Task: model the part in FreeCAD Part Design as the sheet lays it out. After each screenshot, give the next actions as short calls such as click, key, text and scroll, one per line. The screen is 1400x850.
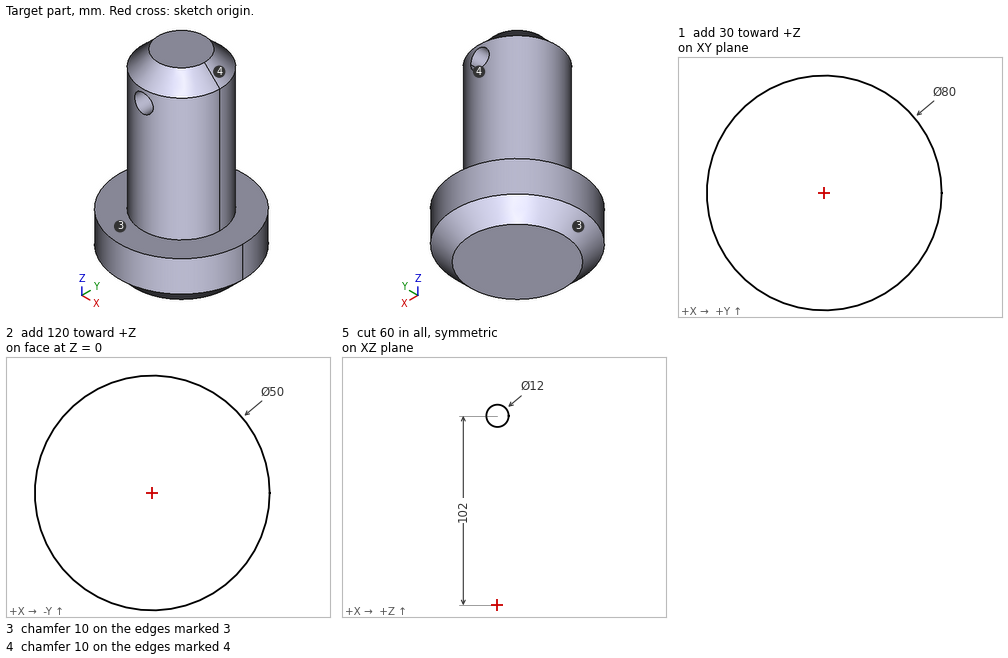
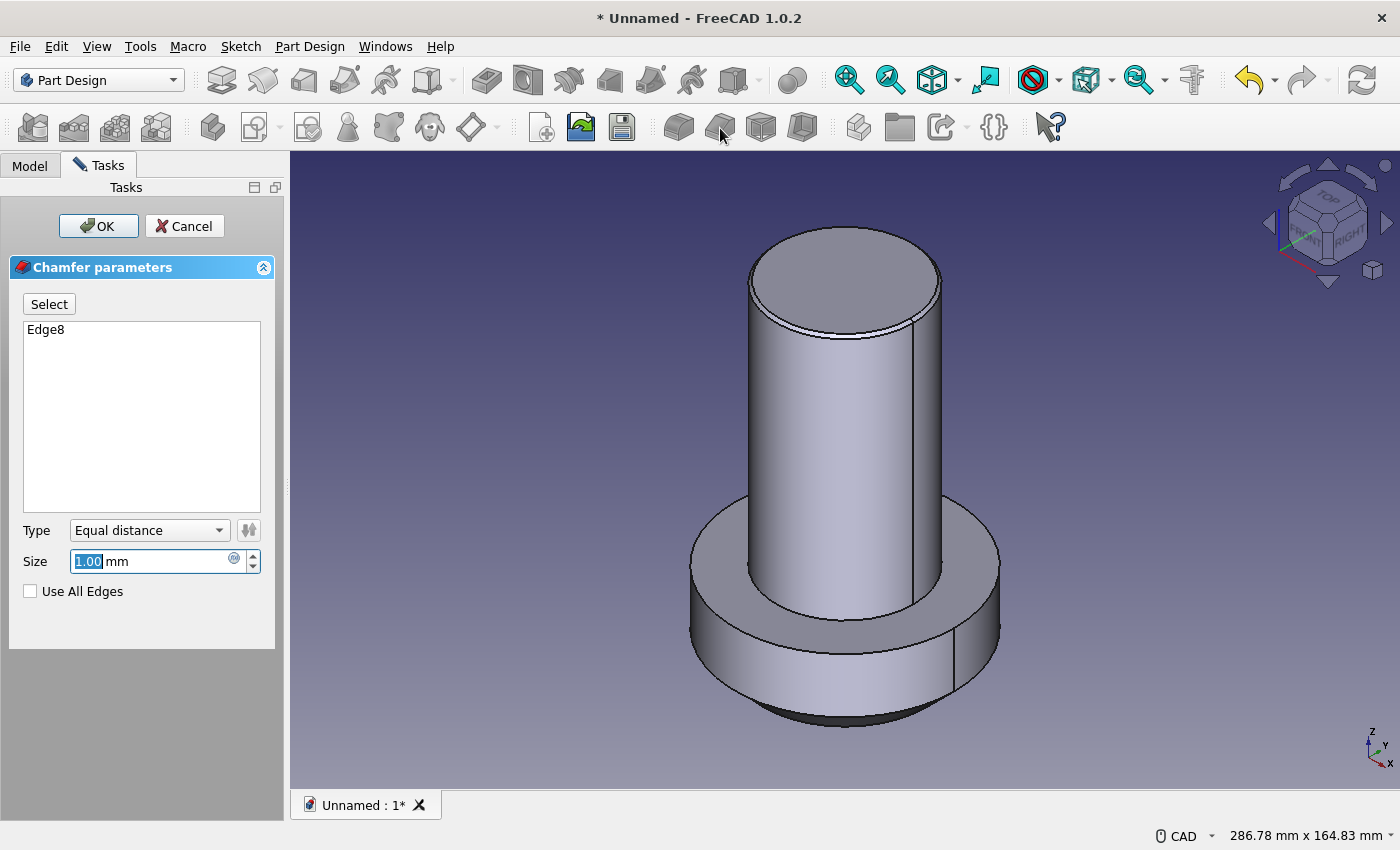
text(10)
key(Tab)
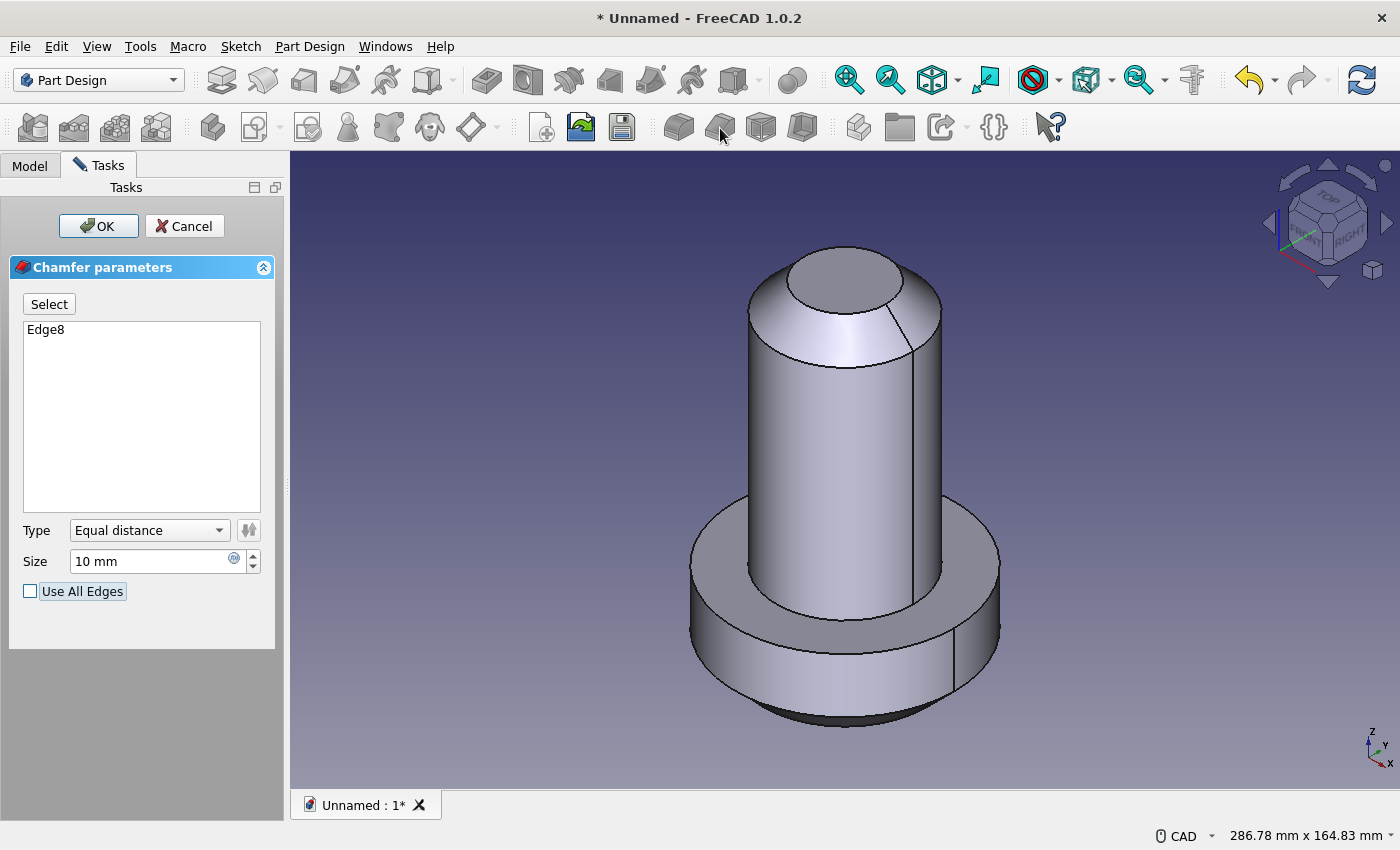
click(99, 226)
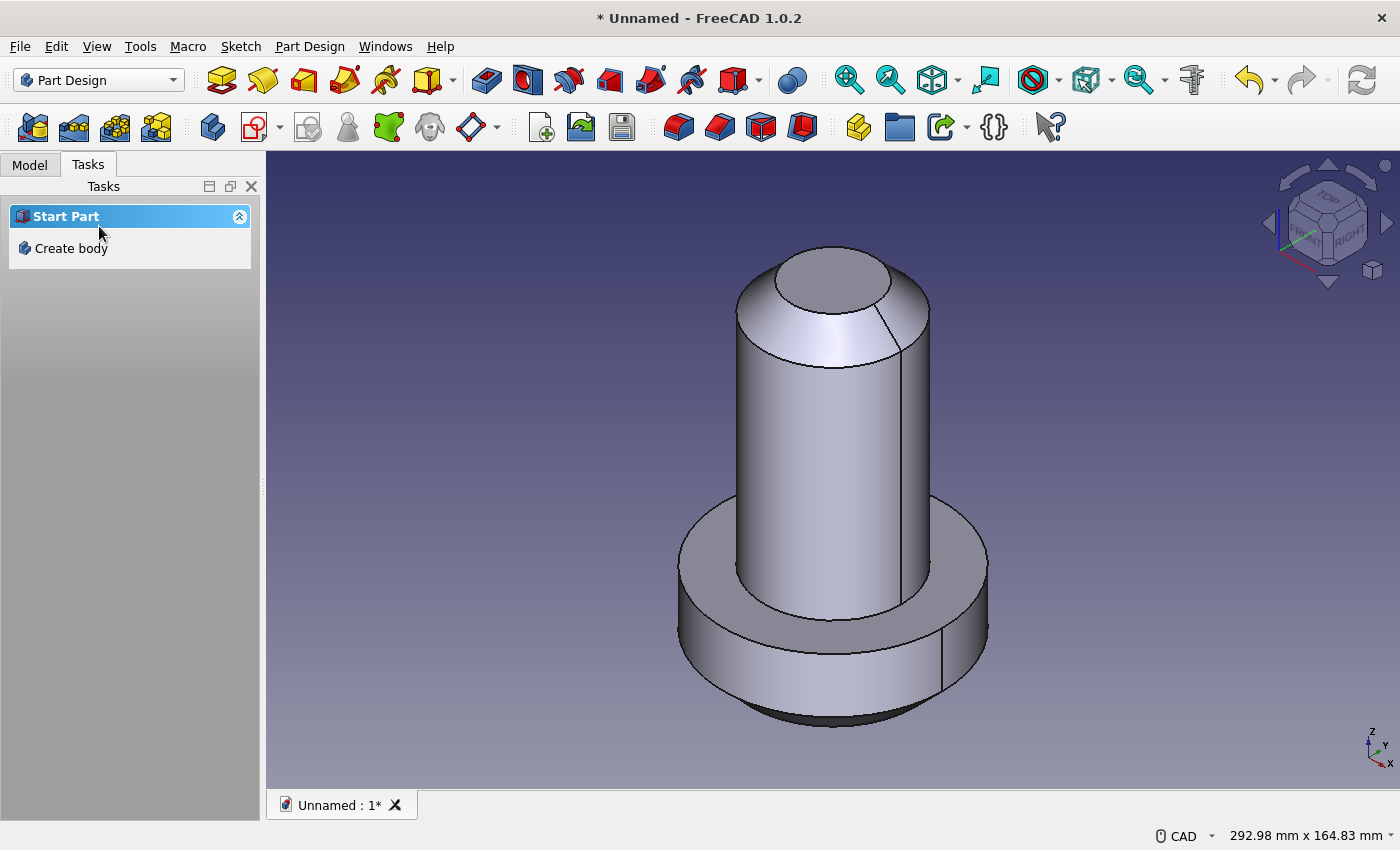
click(254, 128)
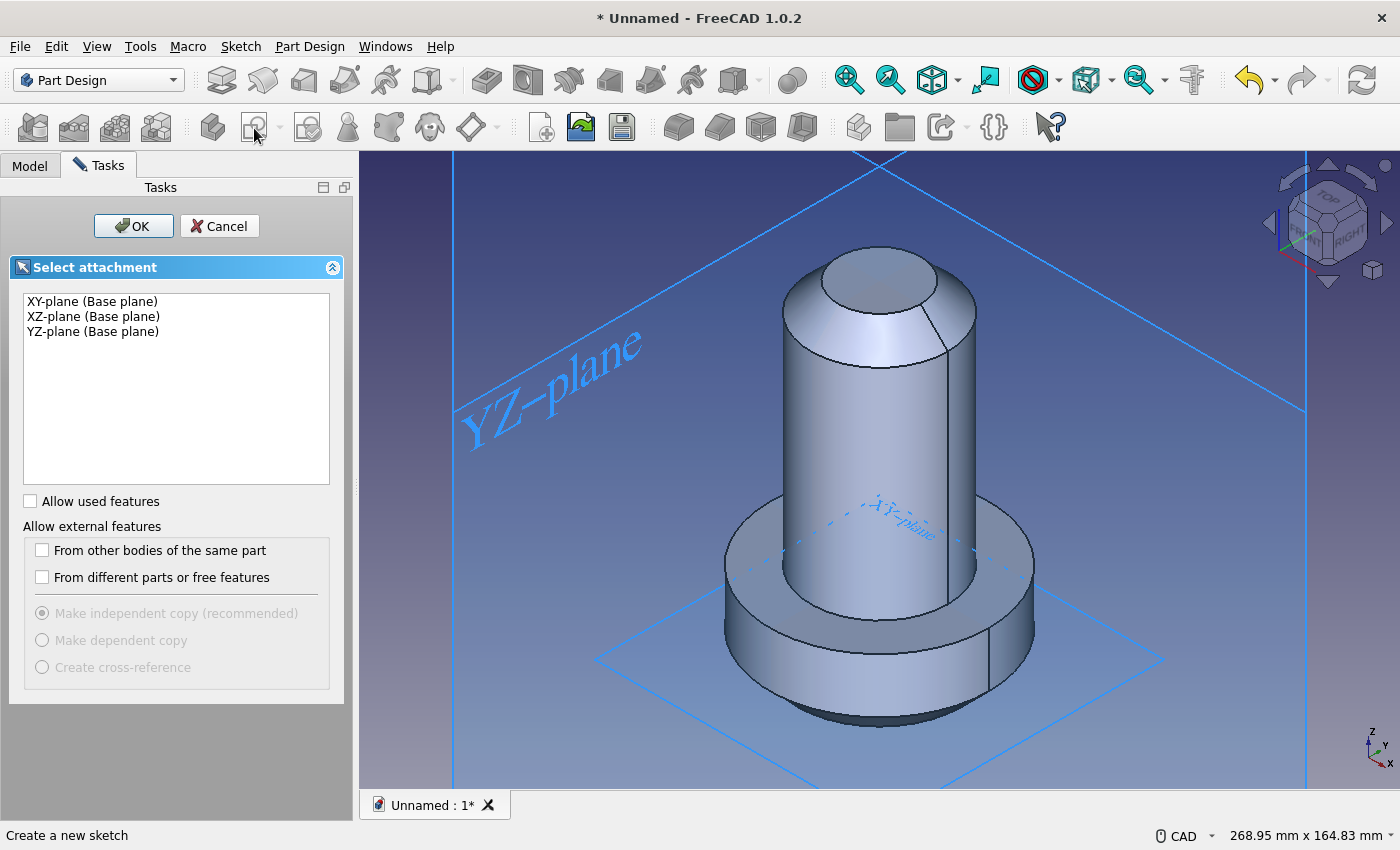
click(84, 316)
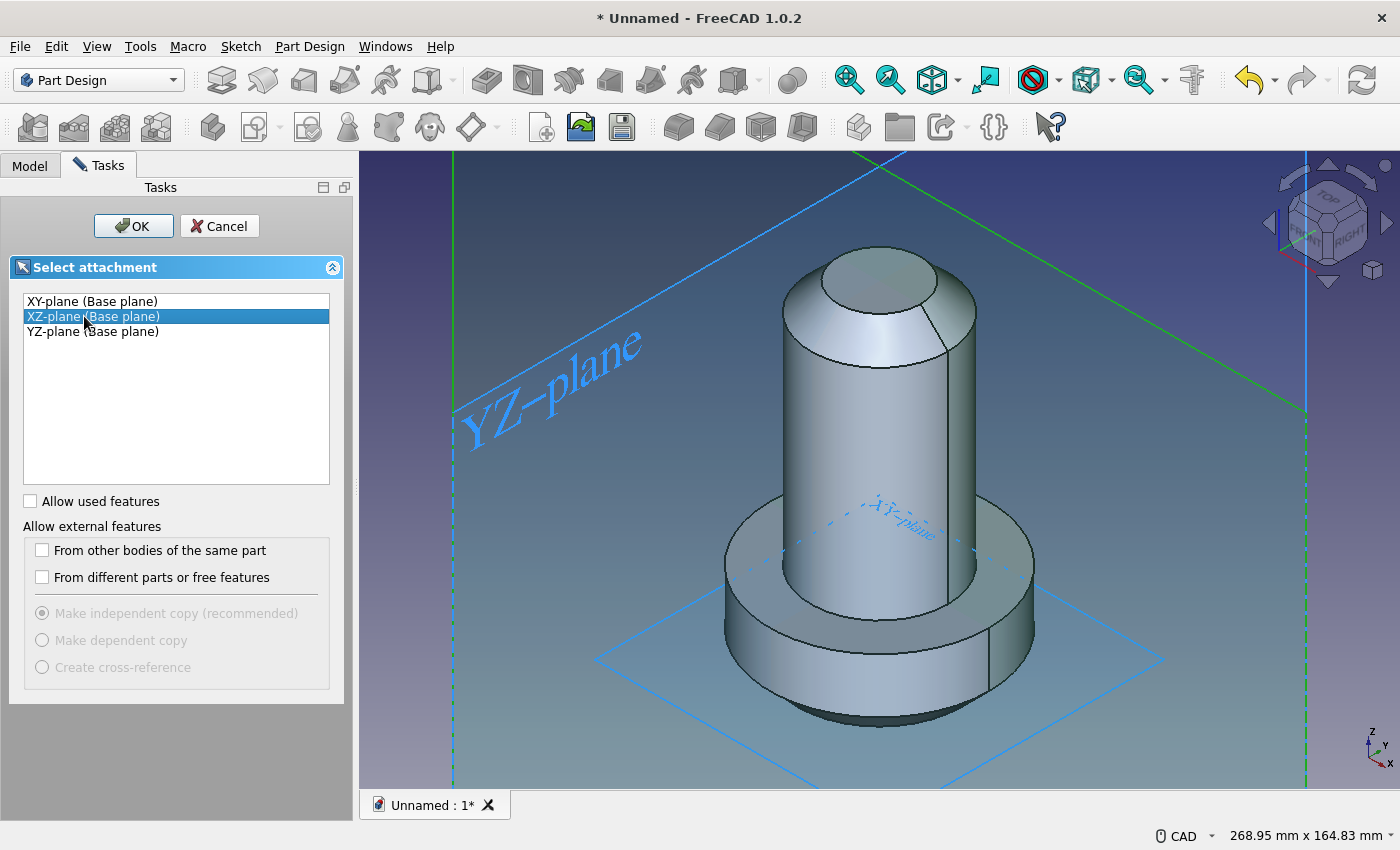
click(134, 226)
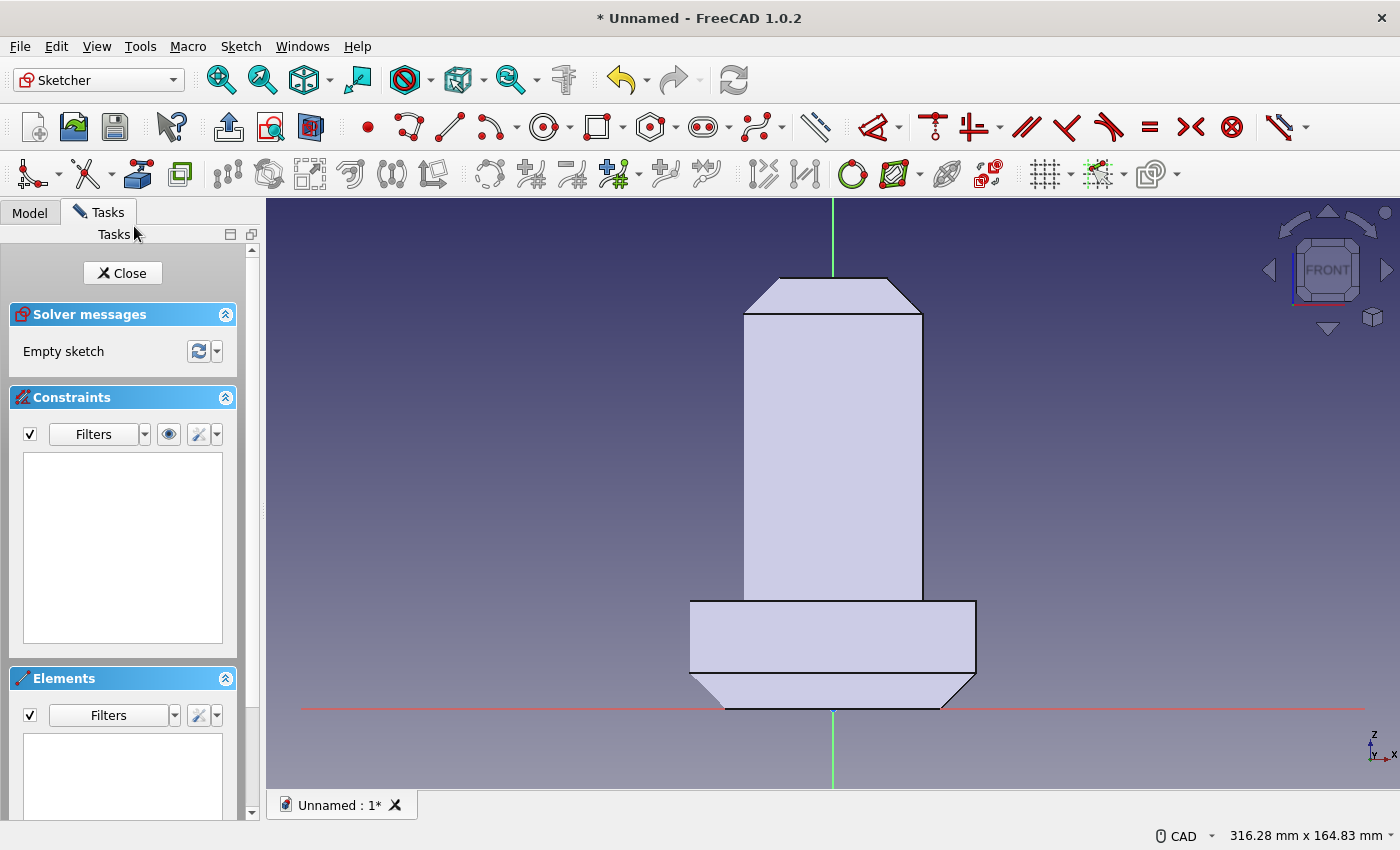
click(311, 128)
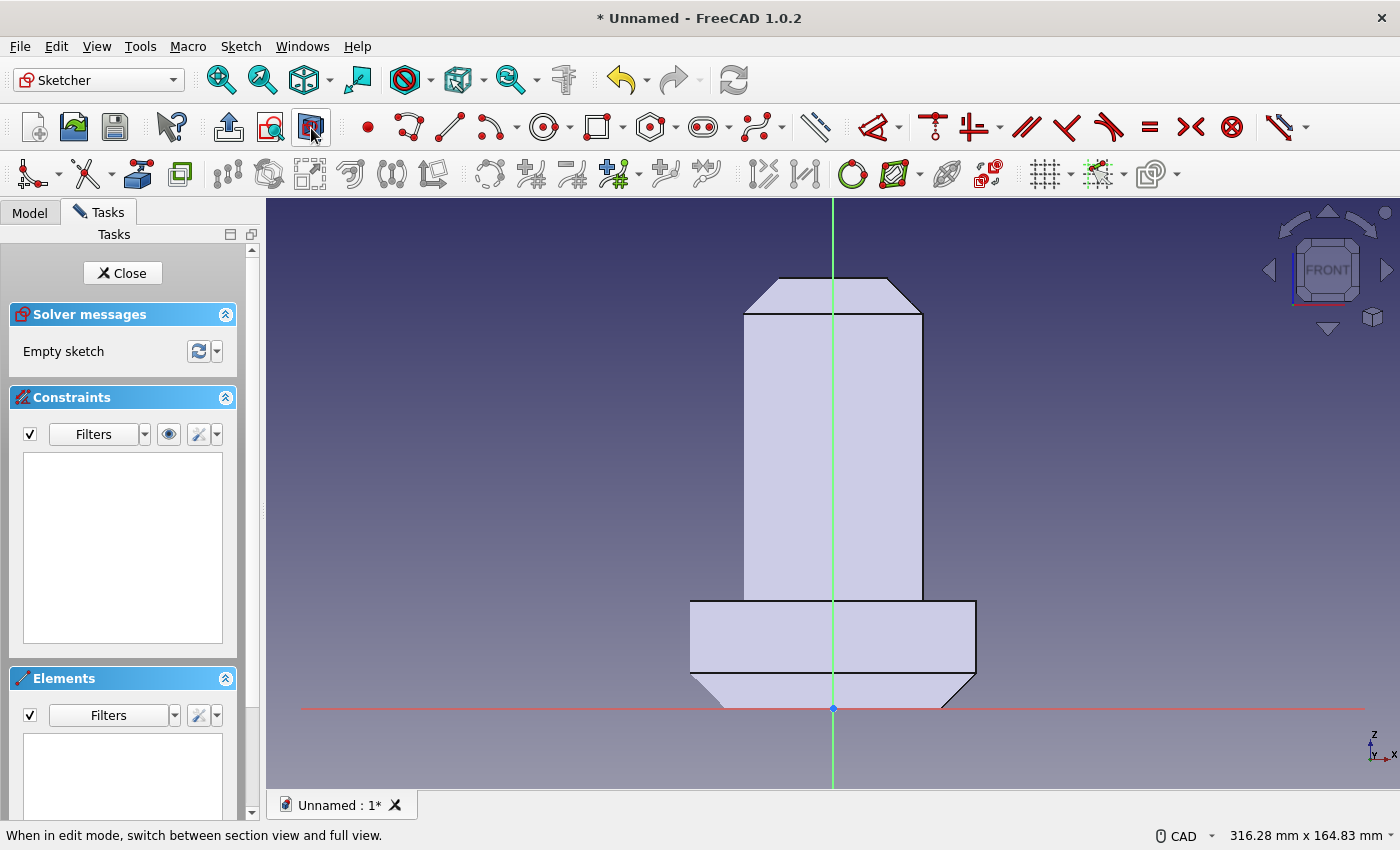
scroll(842, 324, up, 11)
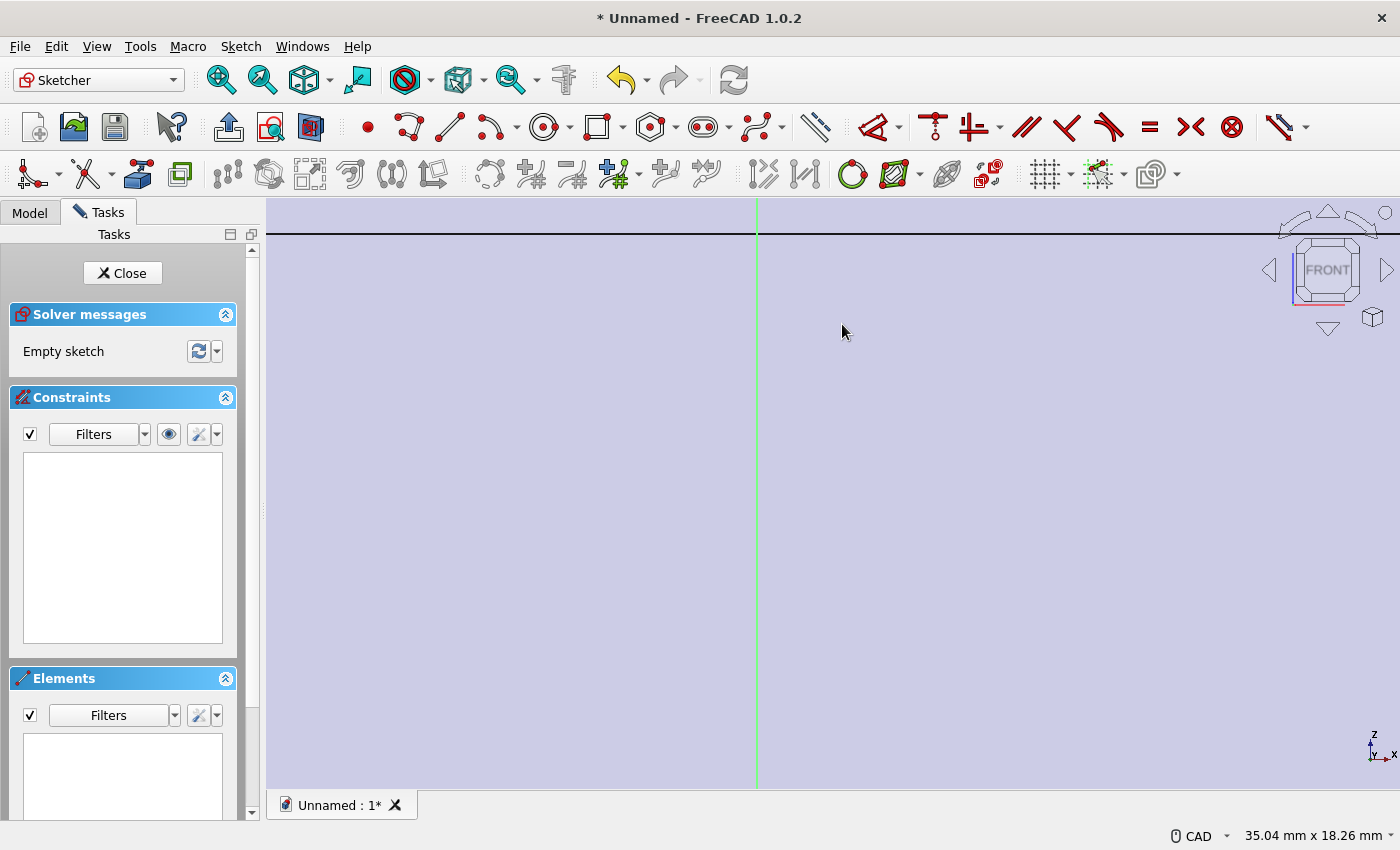
click(544, 128)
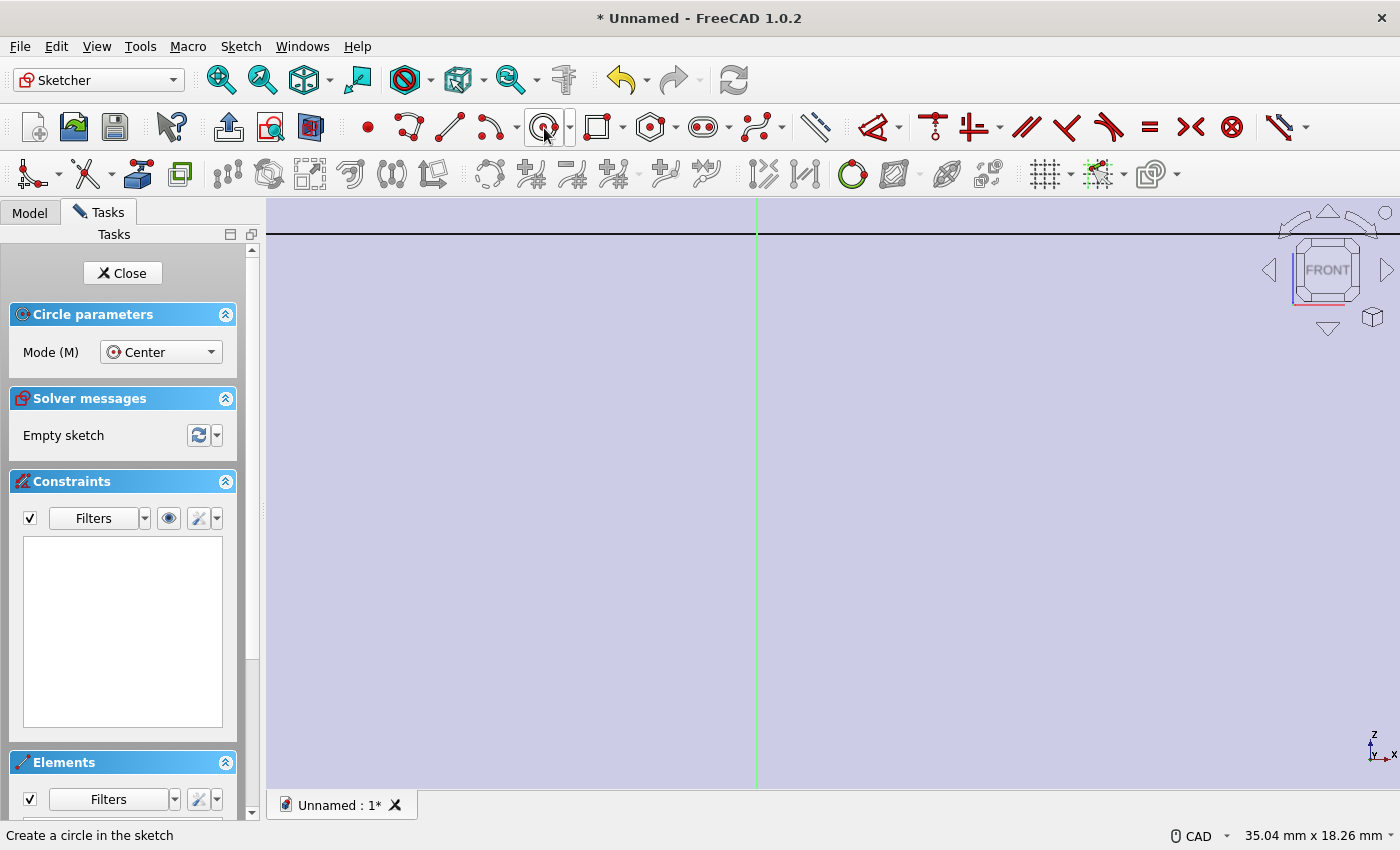
click(757, 493)
click(894, 356)
key(Escape)